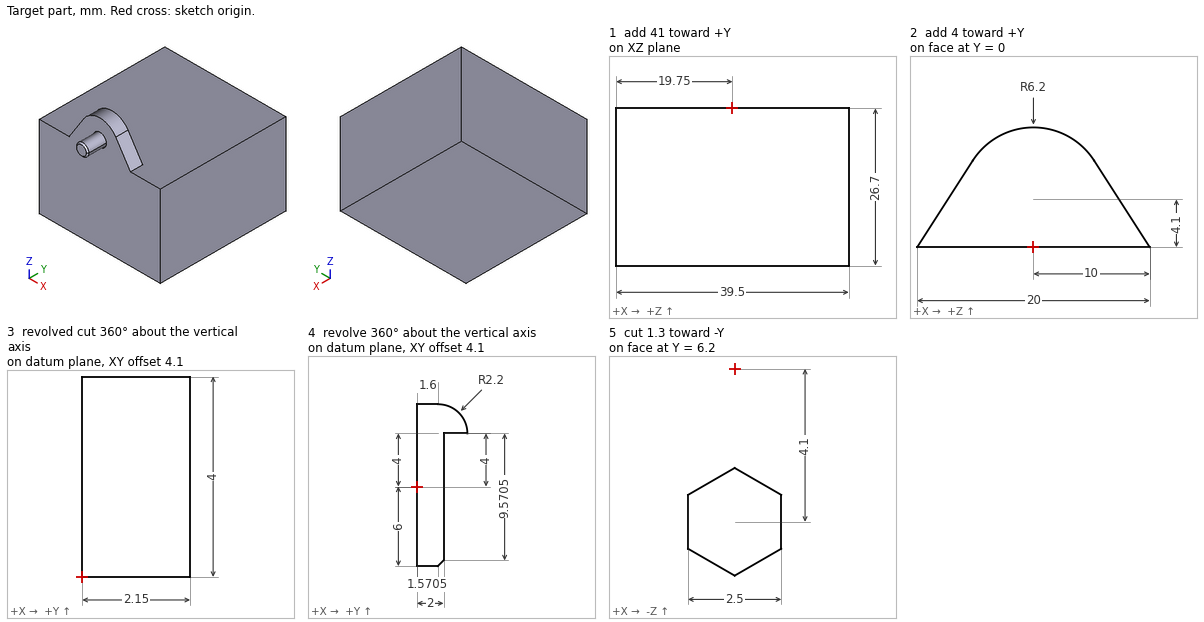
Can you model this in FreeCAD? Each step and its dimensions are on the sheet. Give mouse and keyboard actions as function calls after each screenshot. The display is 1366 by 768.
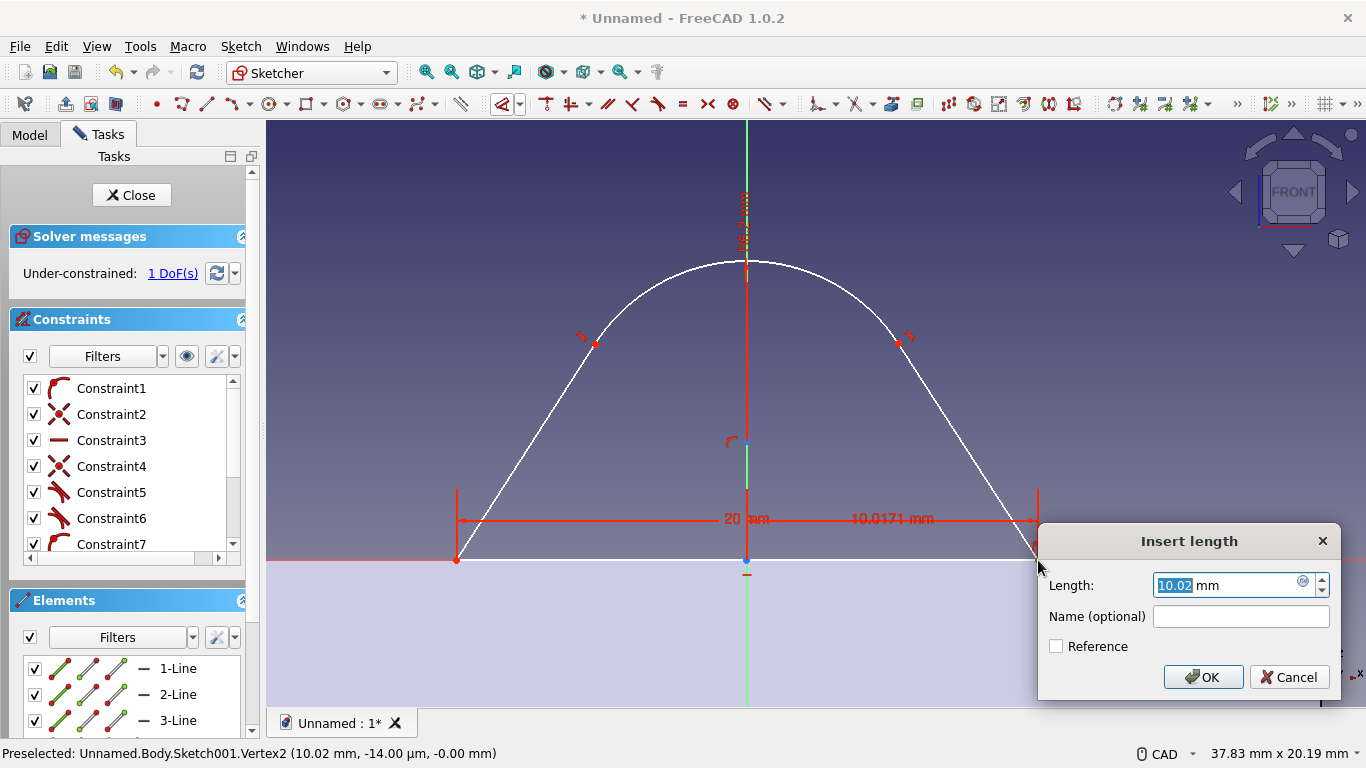
text(10)
key(Return)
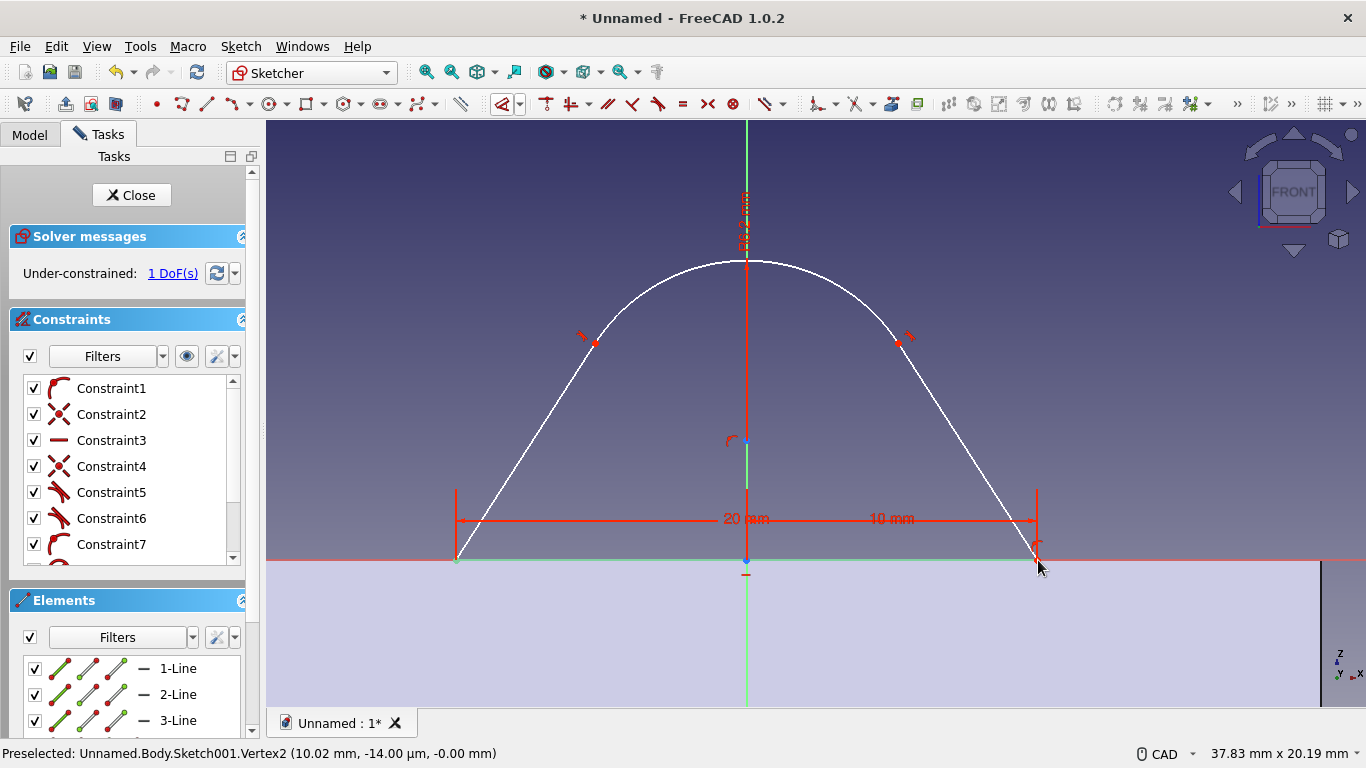
click(747, 441)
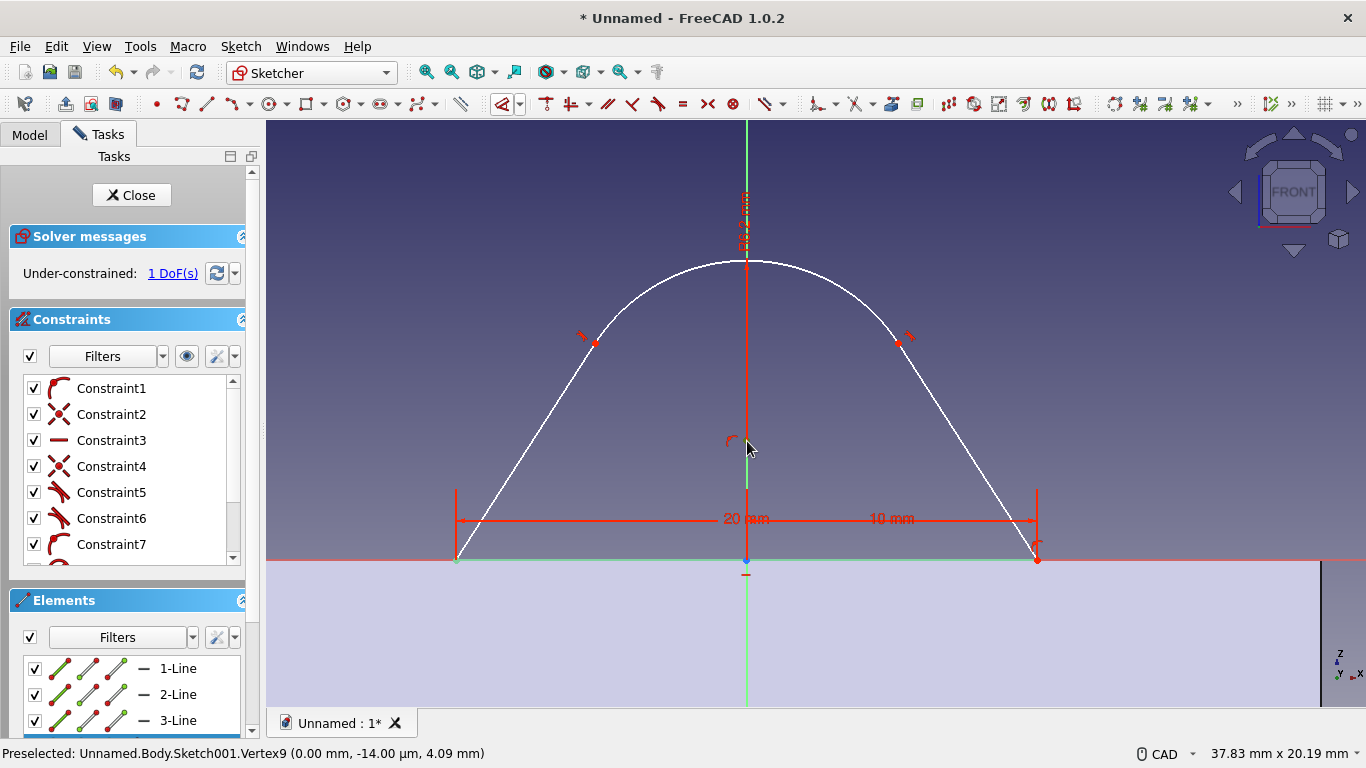
key(i)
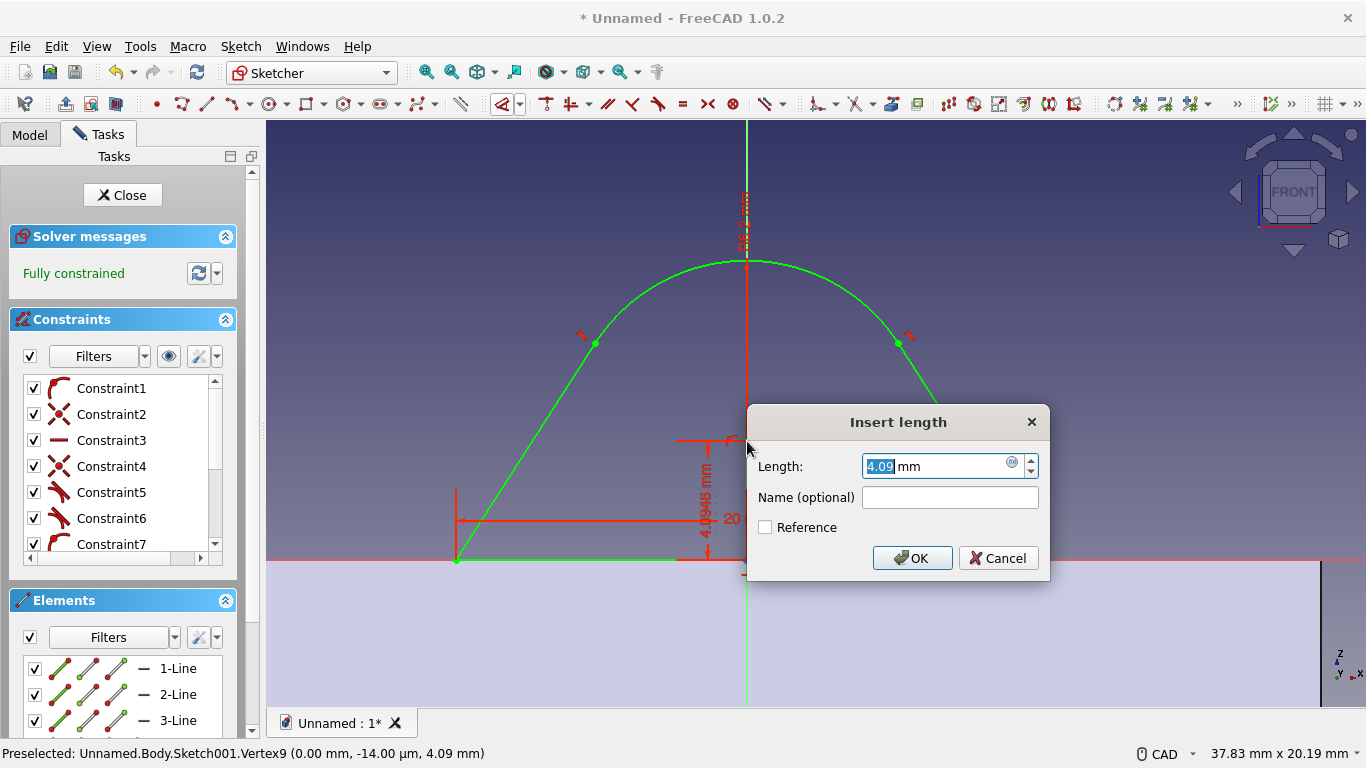
text(4.1)
key(Return)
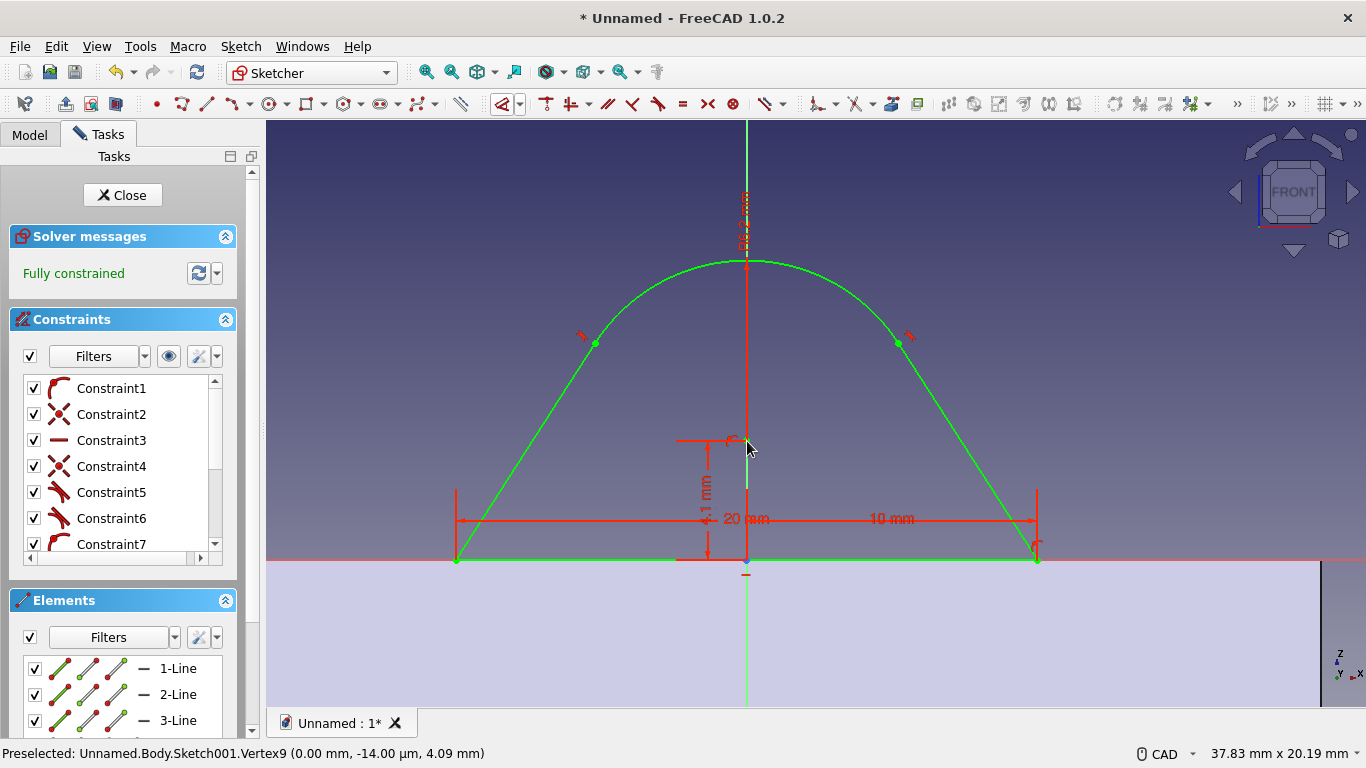
click(123, 195)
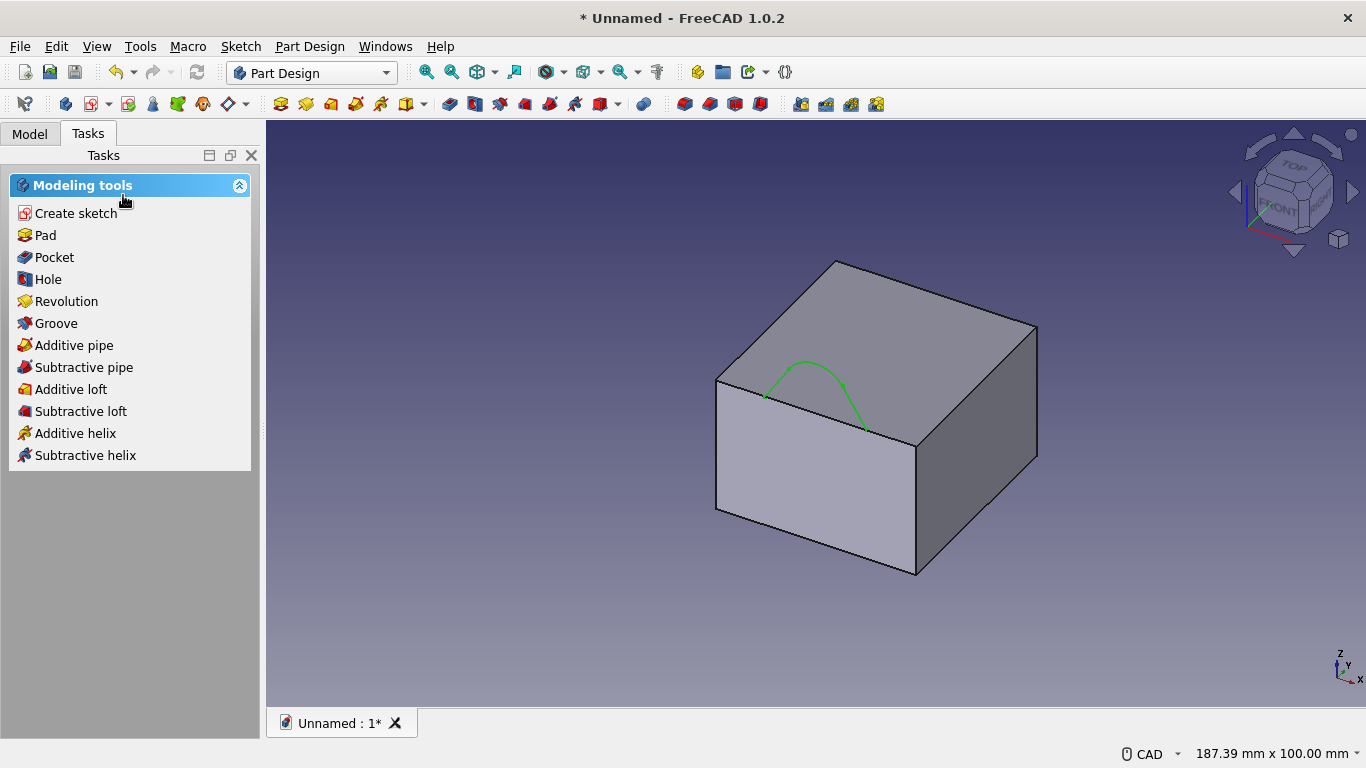
click(281, 104)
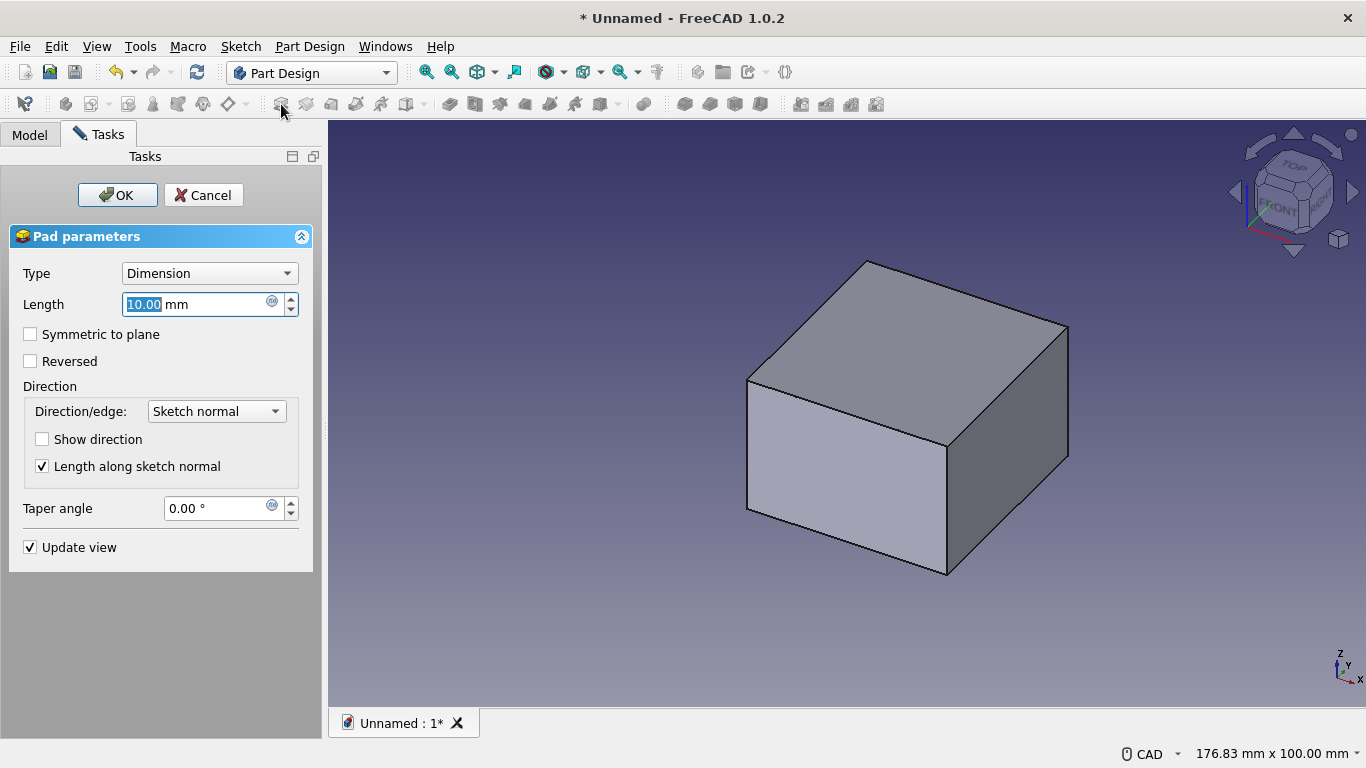
text(4)
key(Tab)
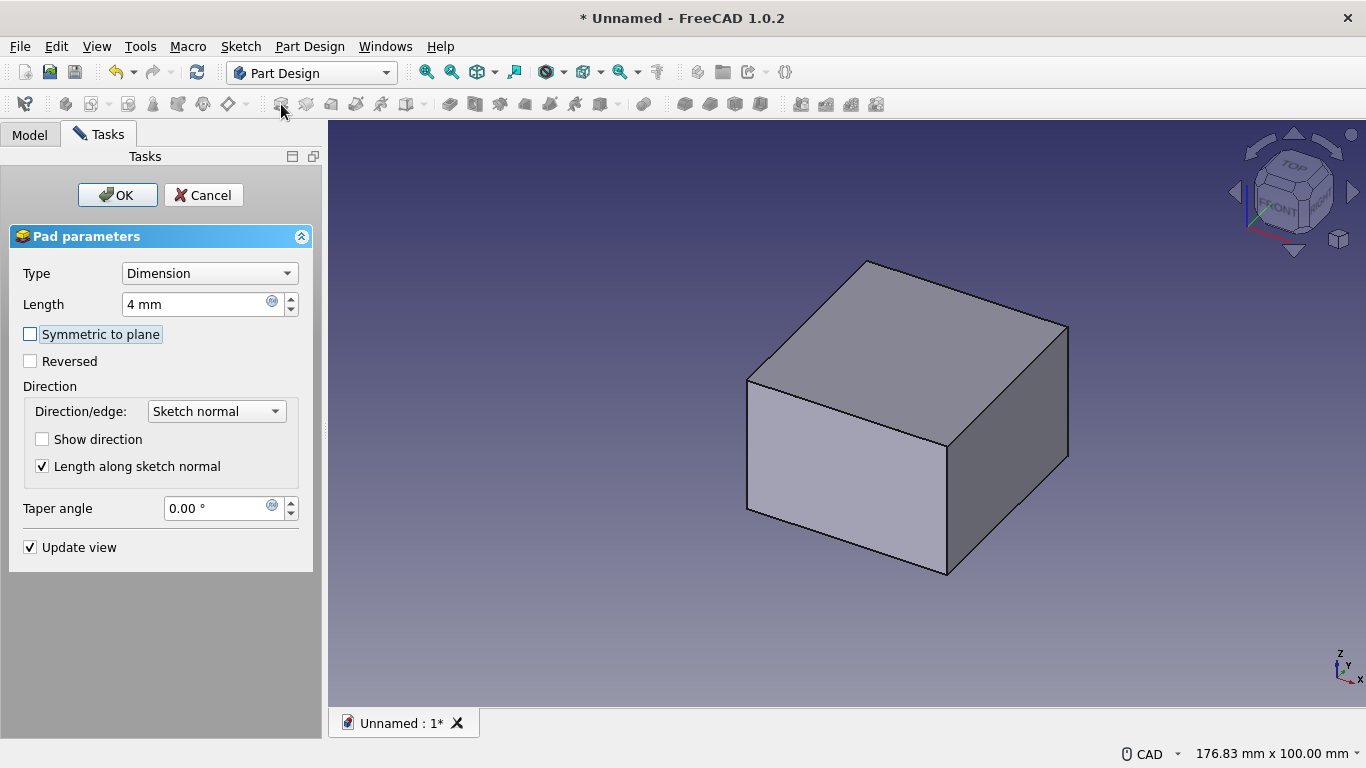
click(31, 361)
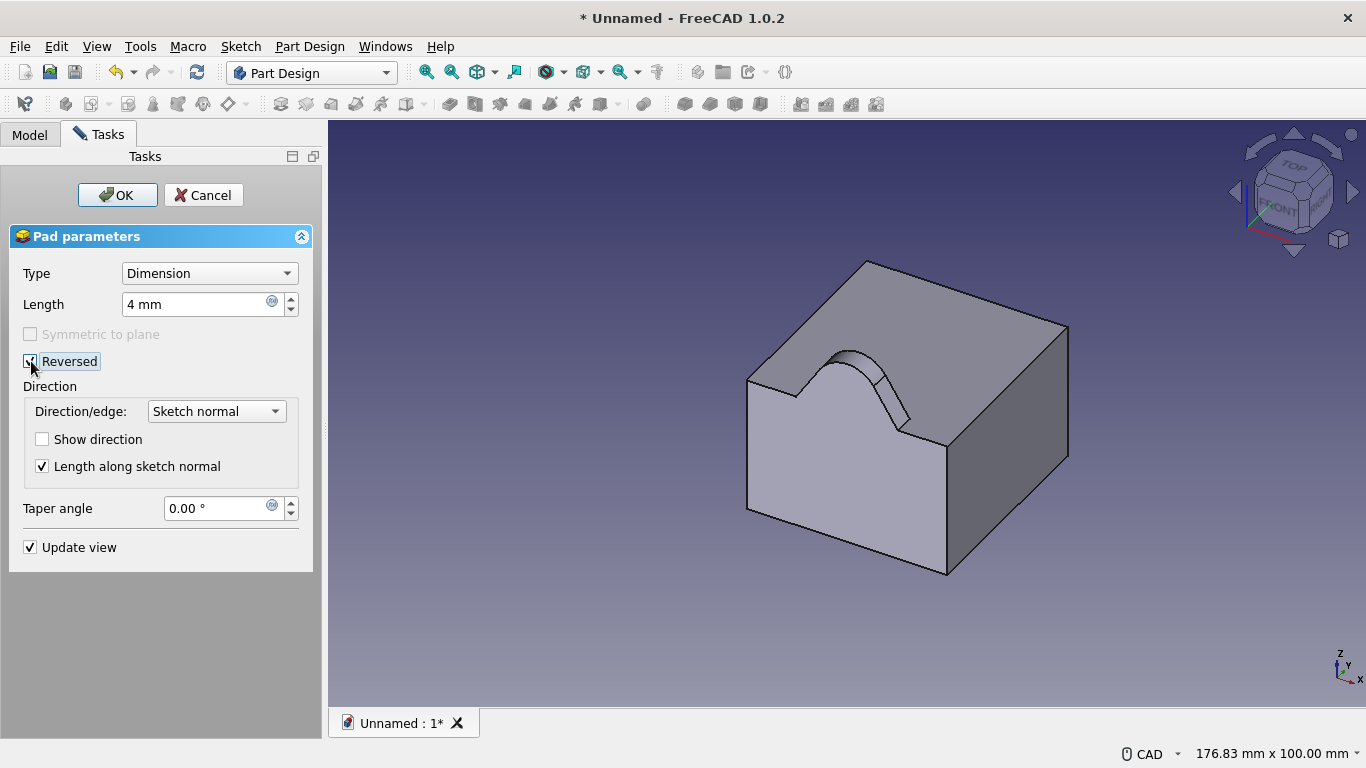
click(118, 195)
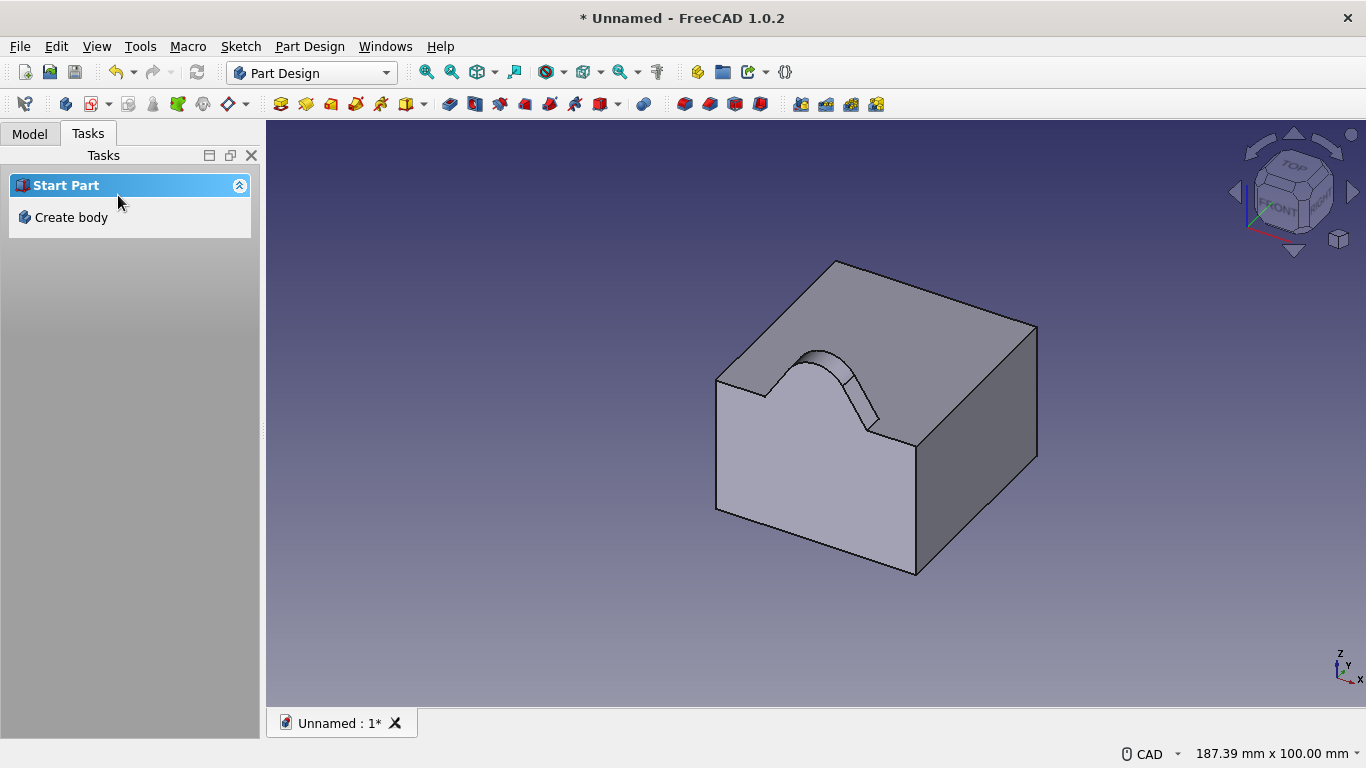
click(30, 134)